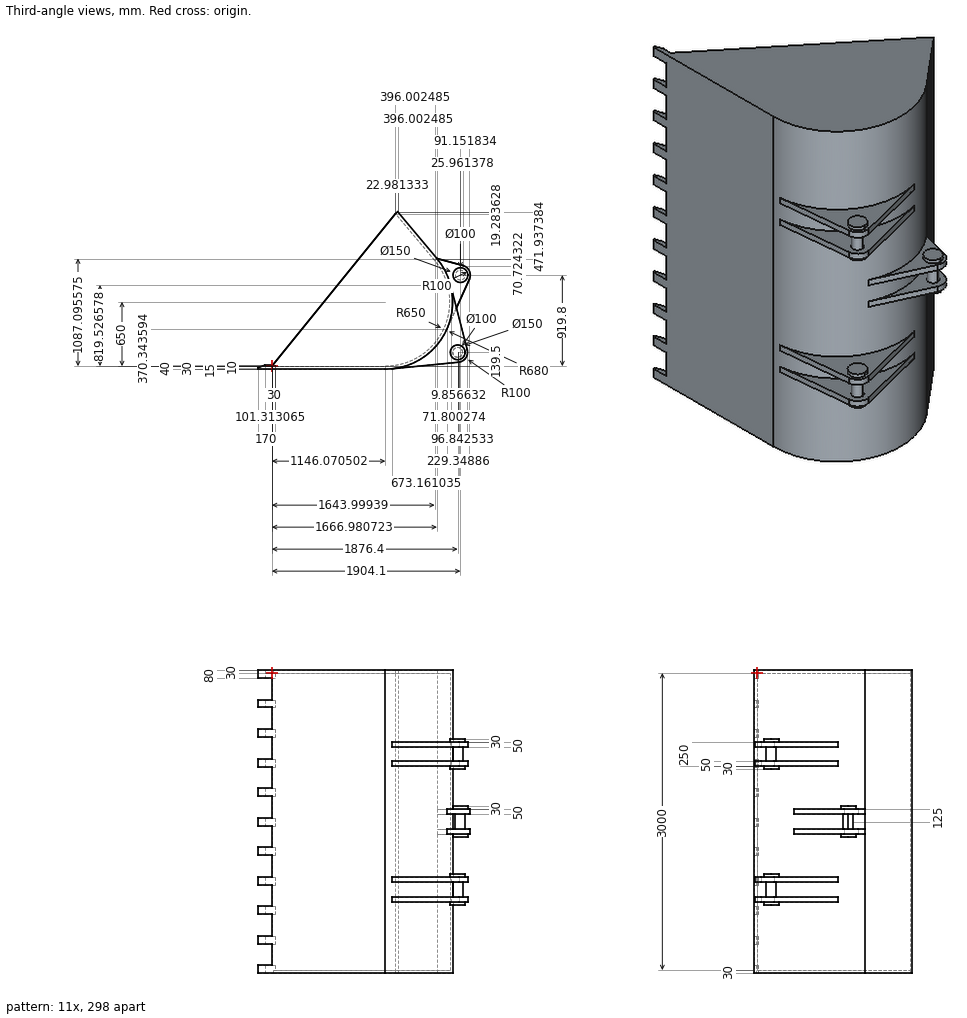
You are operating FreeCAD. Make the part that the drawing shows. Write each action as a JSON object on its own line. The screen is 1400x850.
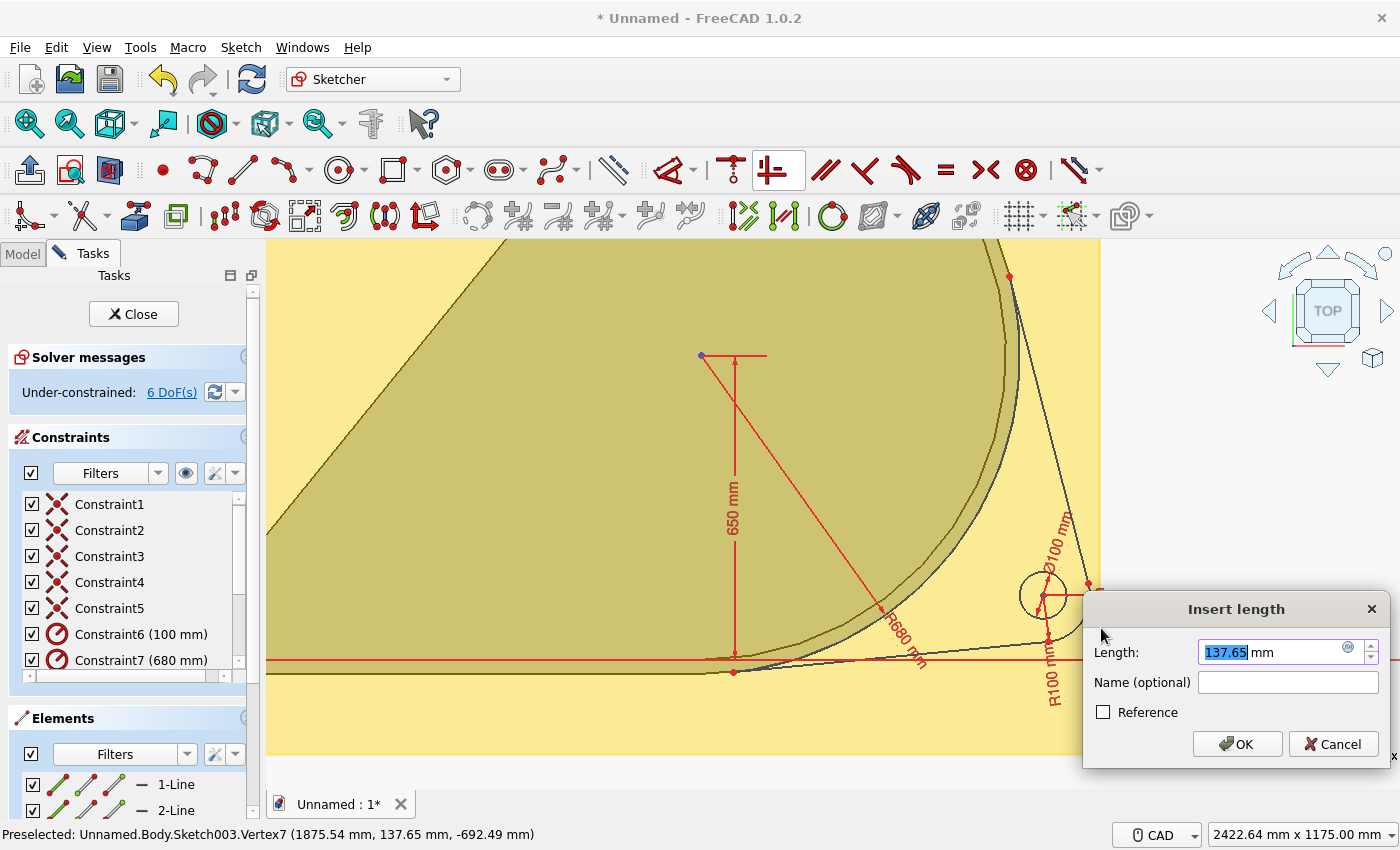
{"action": "type", "text": "139.5"}
{"action": "key", "text": "Return"}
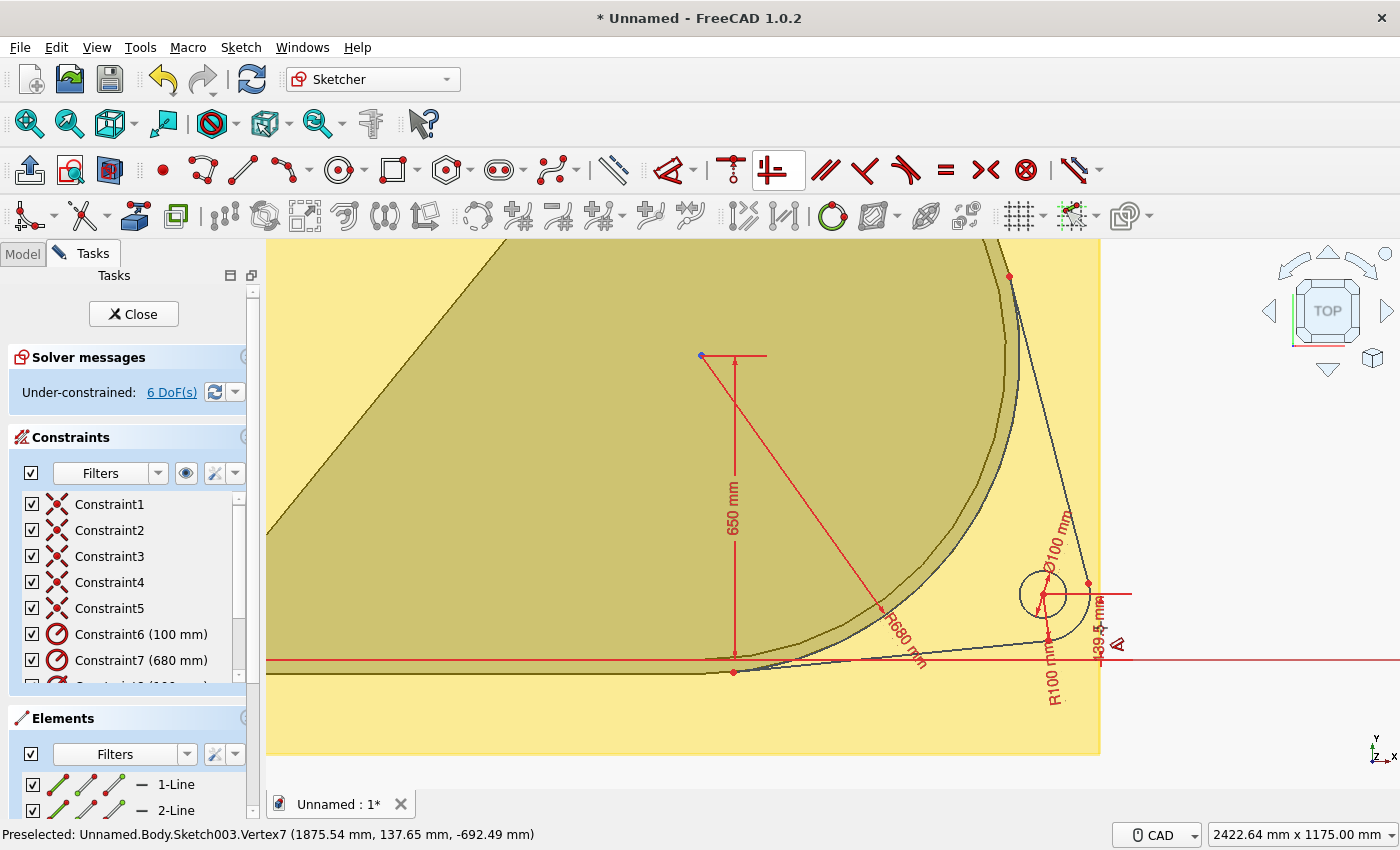
{"action": "left_click", "coordinate": [1043, 594]}
{"action": "left_click", "coordinate": [669, 694]}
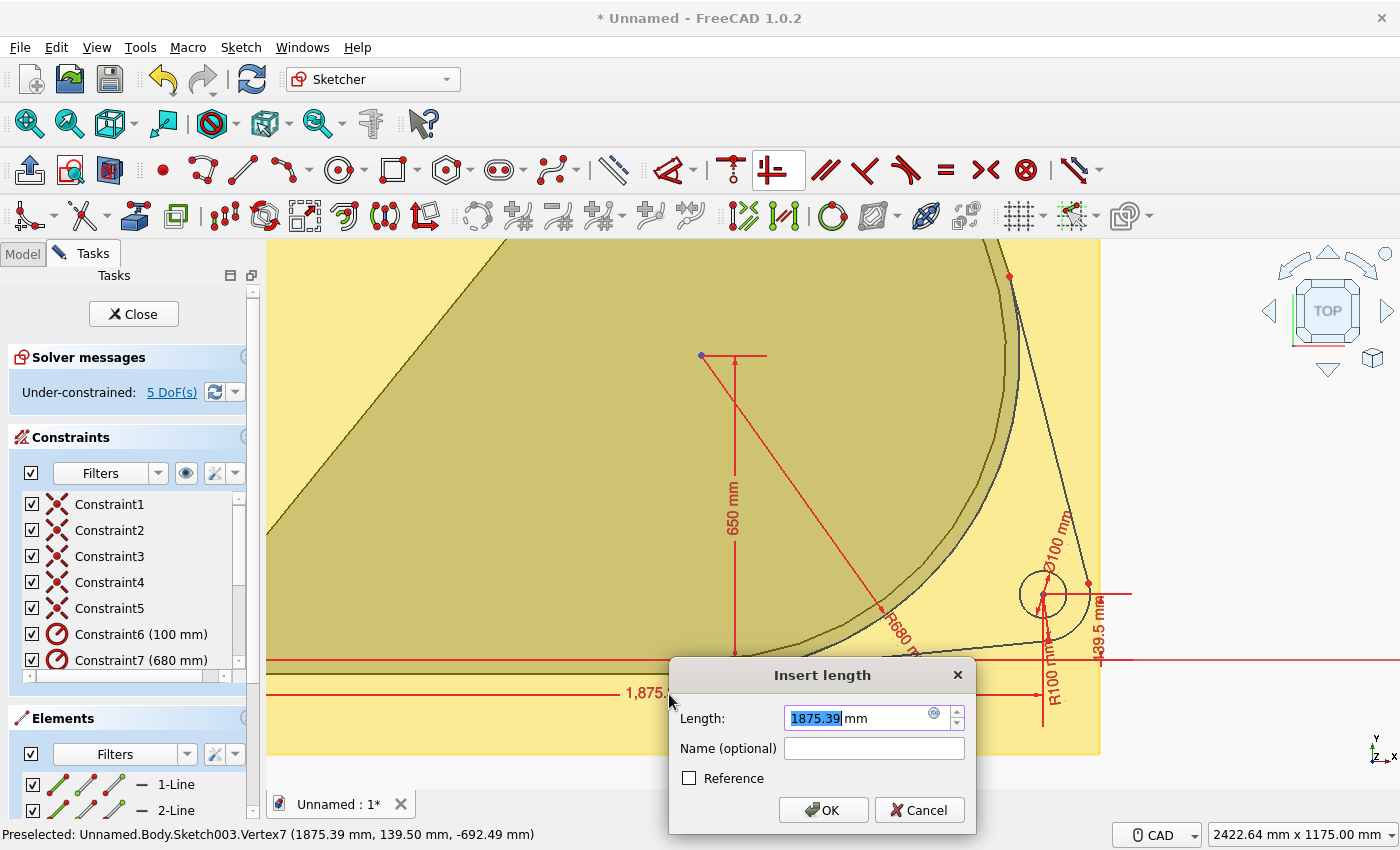
{"action": "type", "text": "1876.4"}
{"action": "key", "text": "Return"}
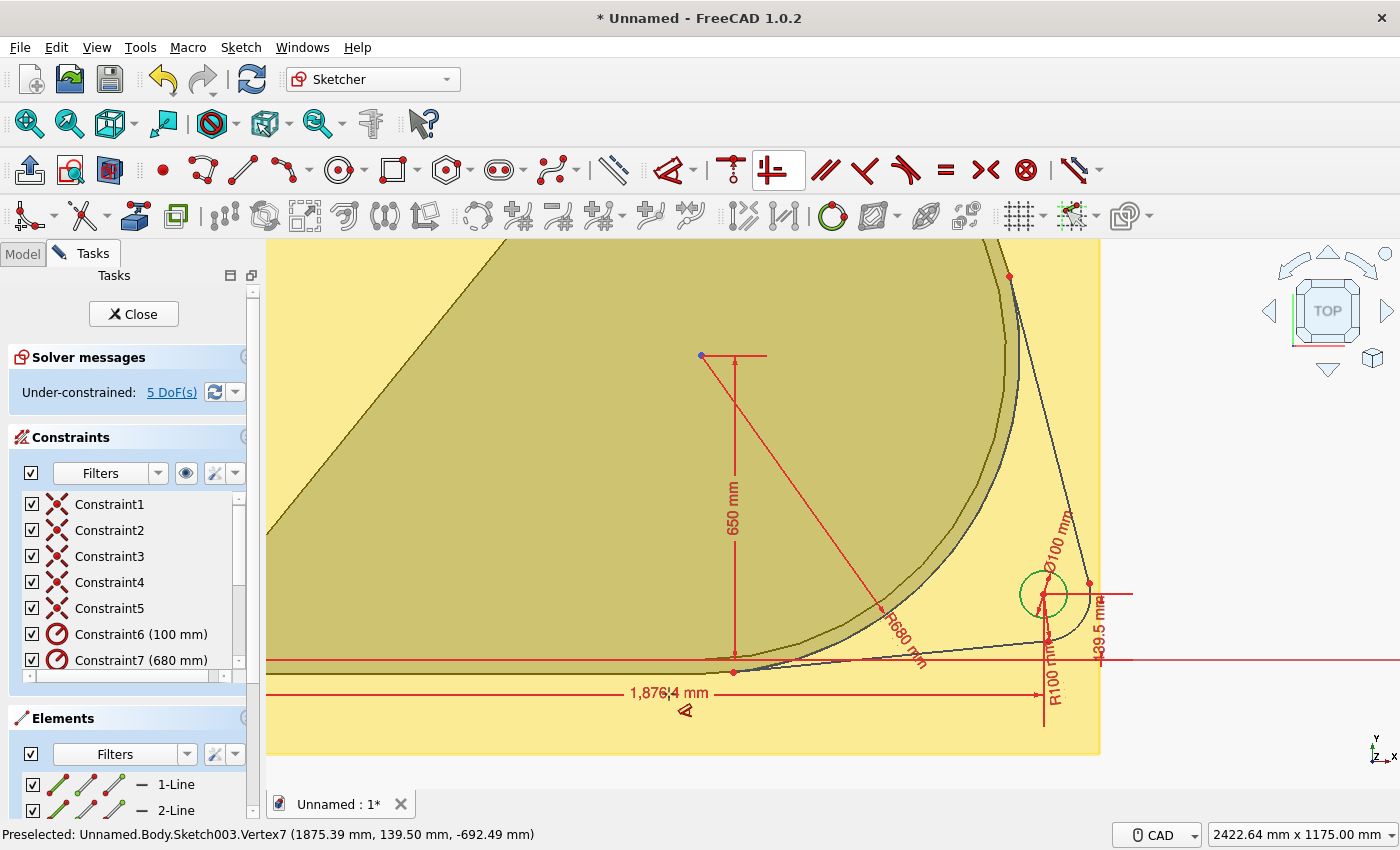
{"action": "scroll", "coordinate": [1048, 641], "scroll_direction": "up", "scroll_amount": 11}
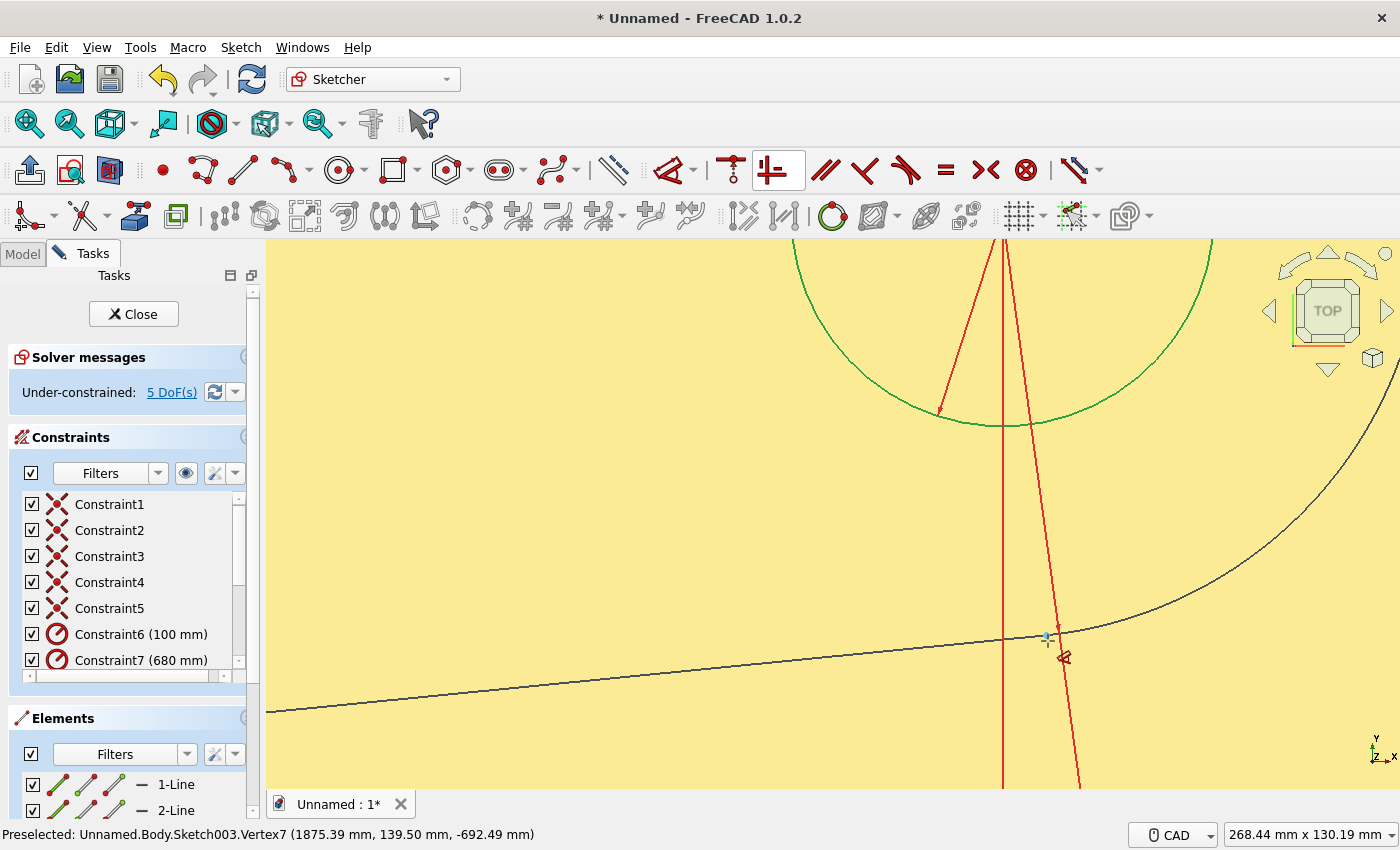
{"action": "left_click", "coordinate": [1047, 635]}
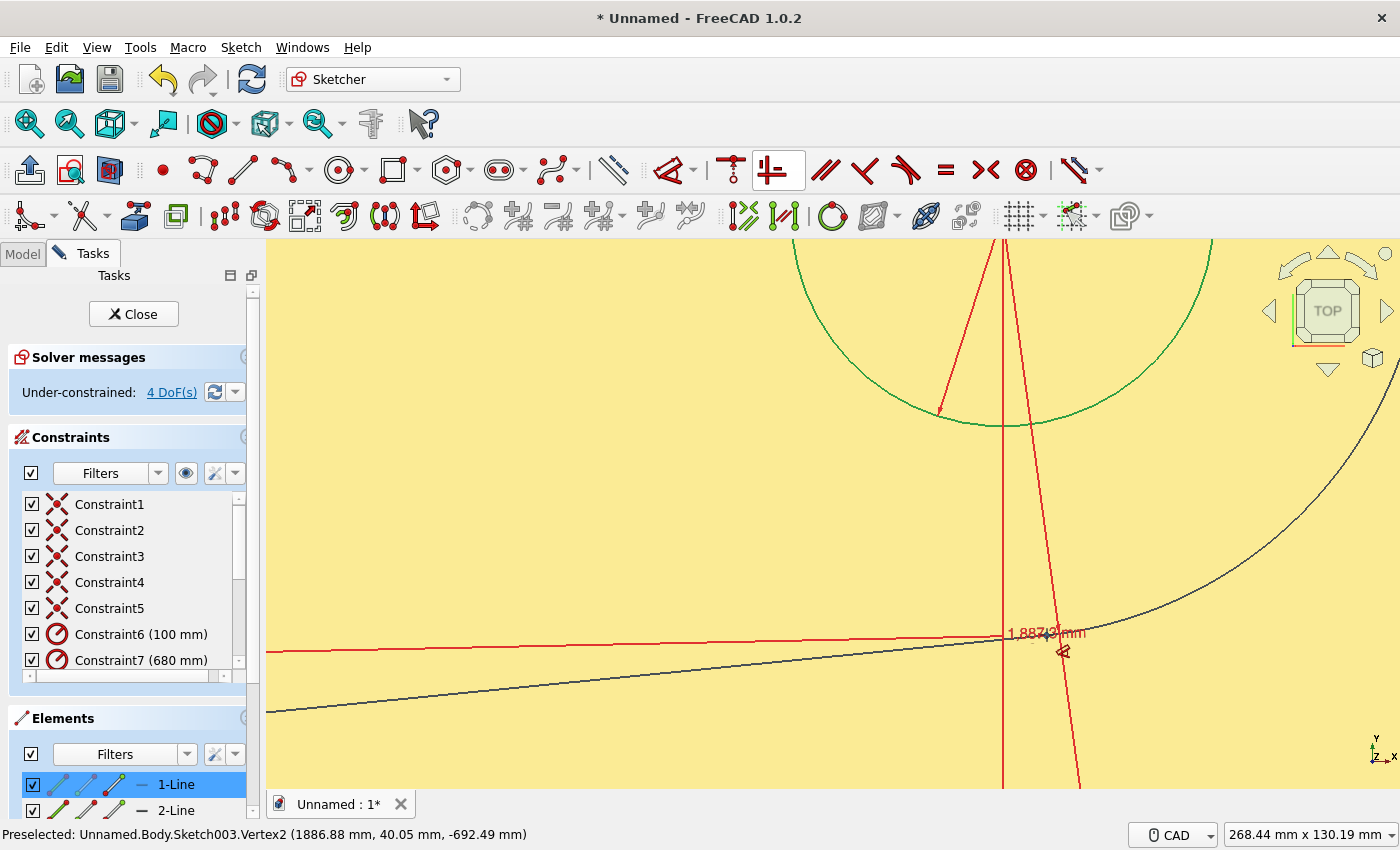
{"action": "scroll", "coordinate": [1047, 625], "scroll_direction": "down", "scroll_amount": 13}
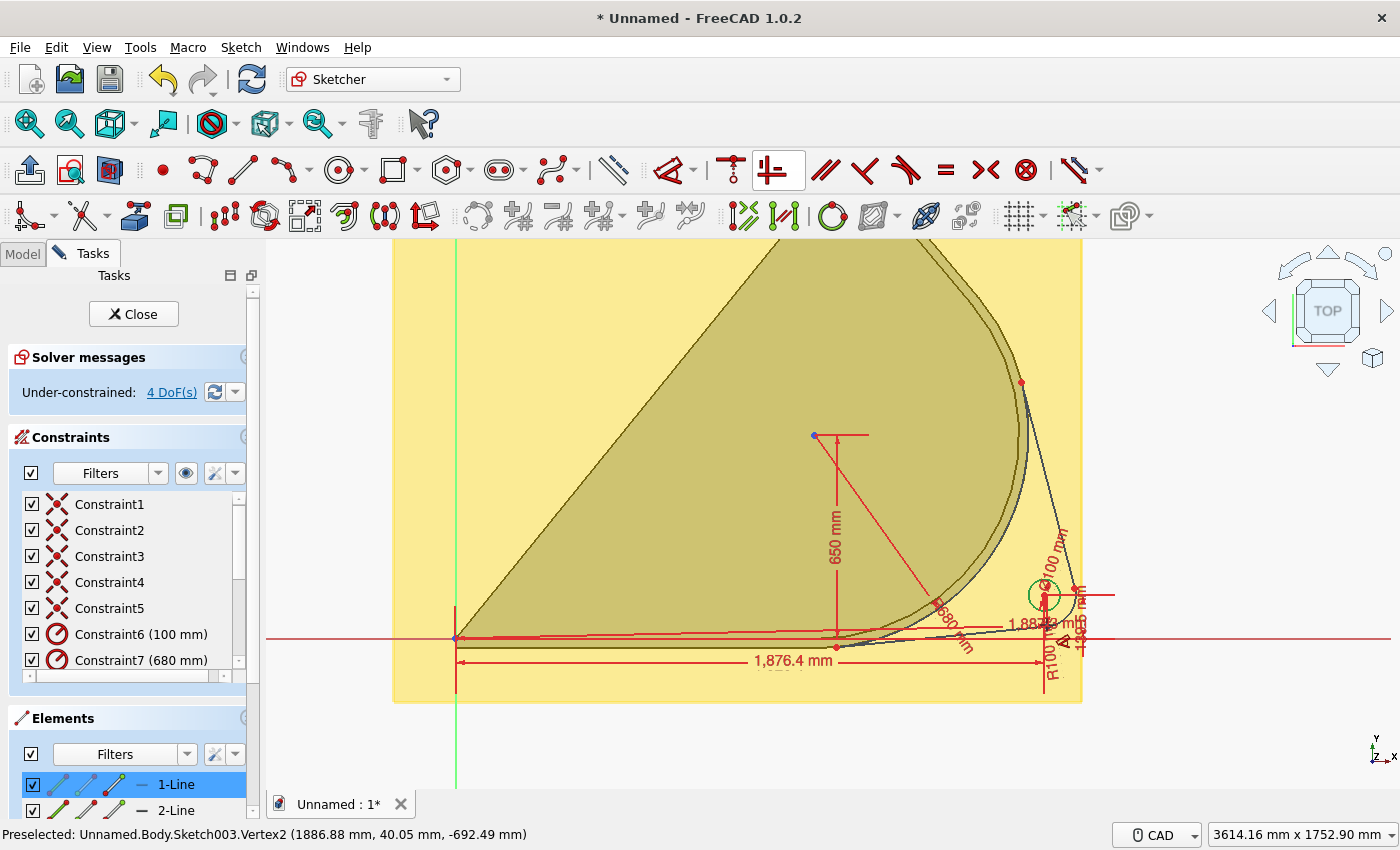
{"action": "scroll", "coordinate": [1044, 595], "scroll_direction": "up", "scroll_amount": 13}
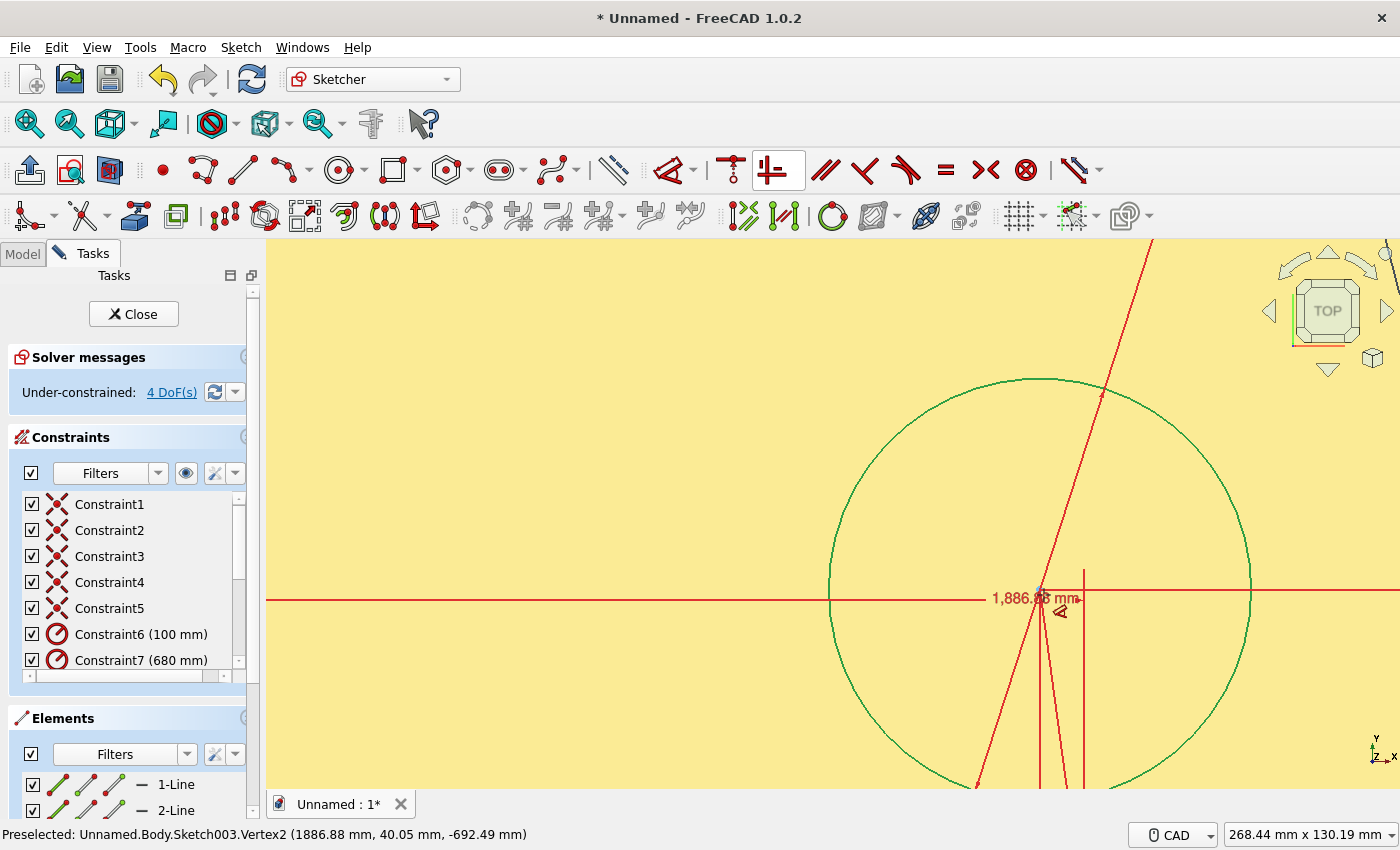
{"action": "left_click", "coordinate": [1040, 590]}
{"action": "left_click", "coordinate": [1062, 556]}